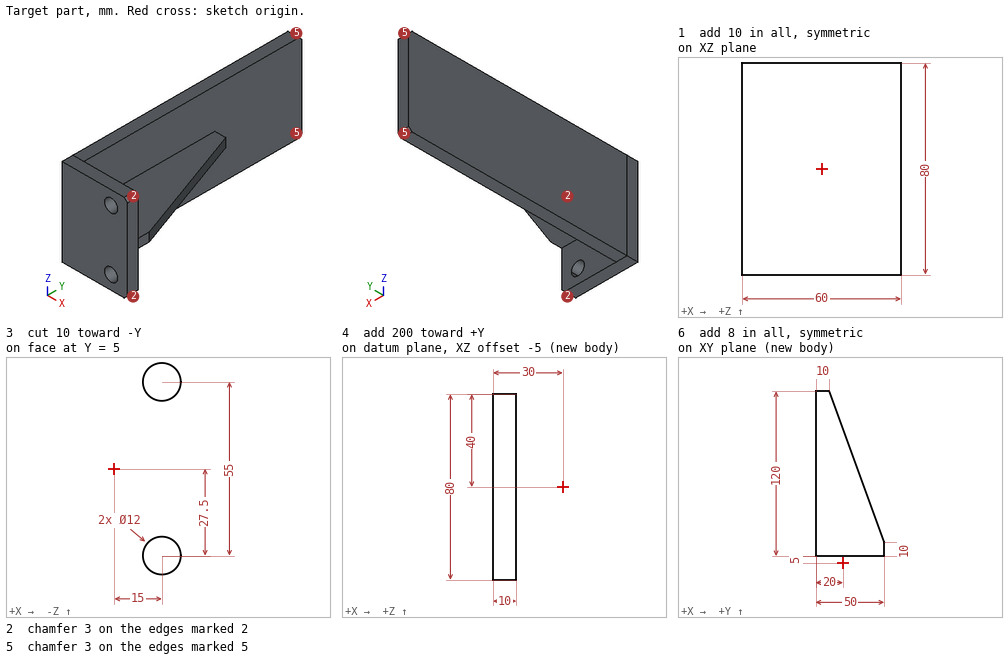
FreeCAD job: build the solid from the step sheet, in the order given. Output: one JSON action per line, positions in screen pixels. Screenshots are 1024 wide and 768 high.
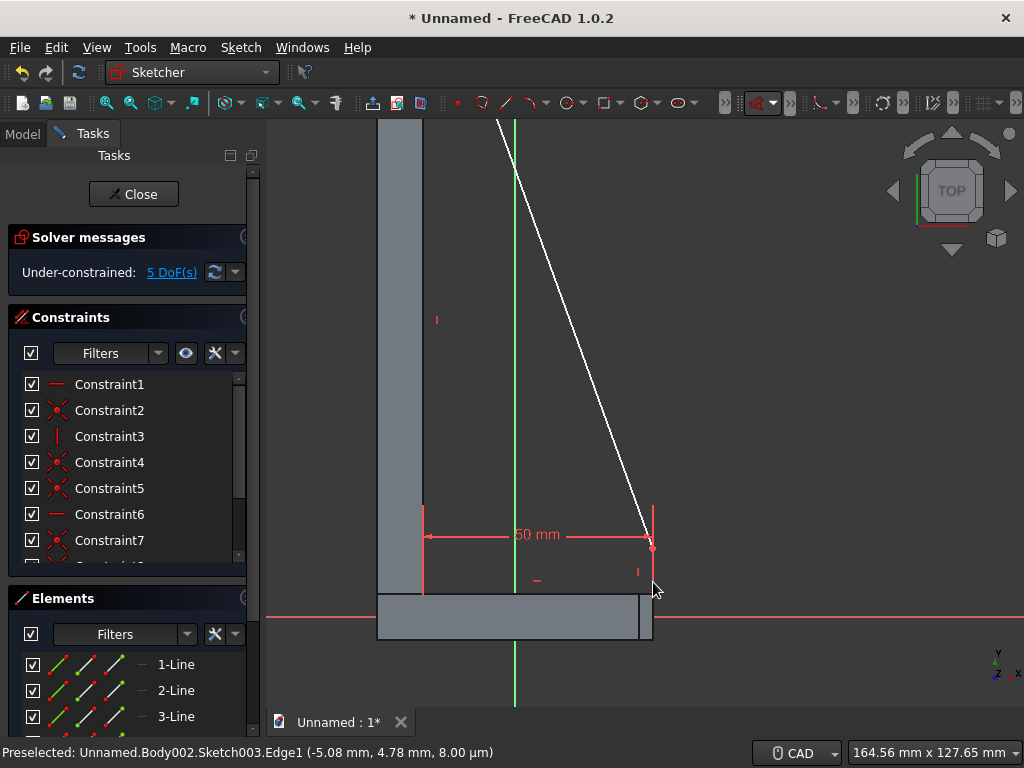
{"action": "left_click", "coordinate": [653, 581]}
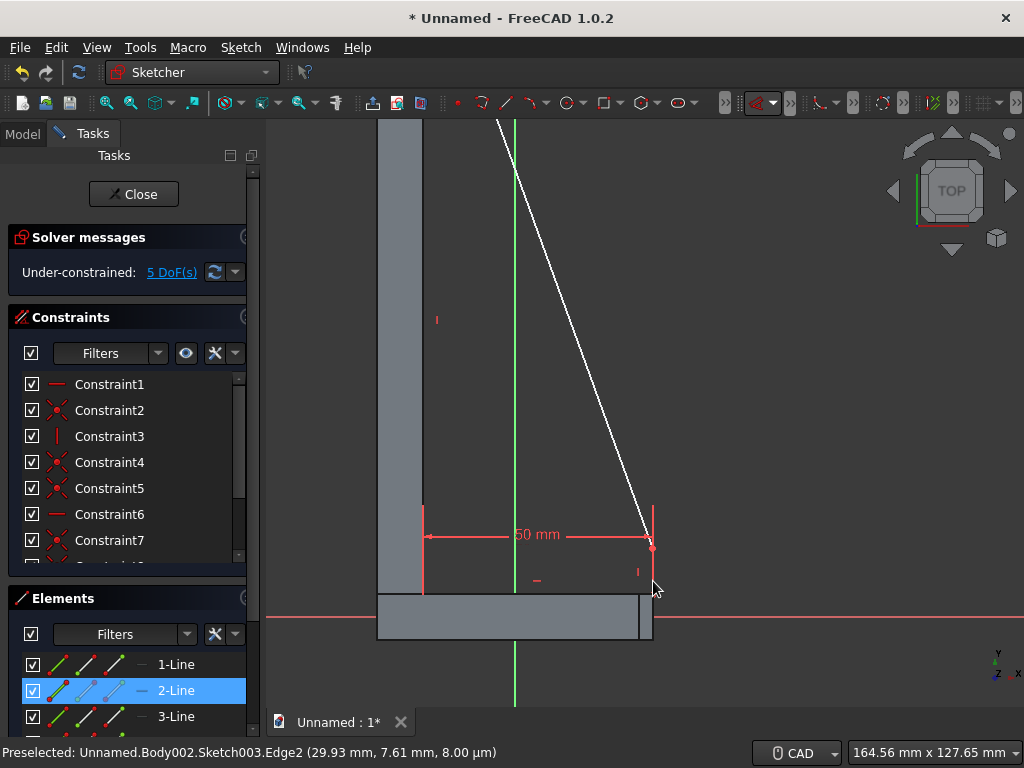
{"action": "left_click", "coordinate": [776, 104]}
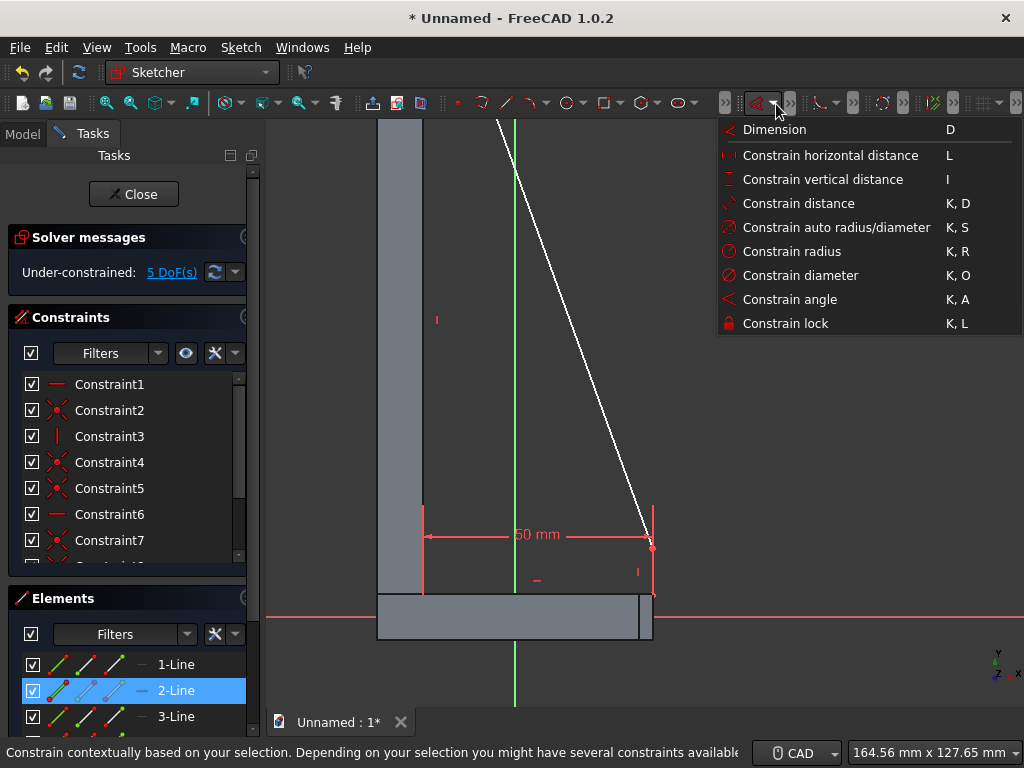
{"action": "left_click", "coordinate": [870, 179]}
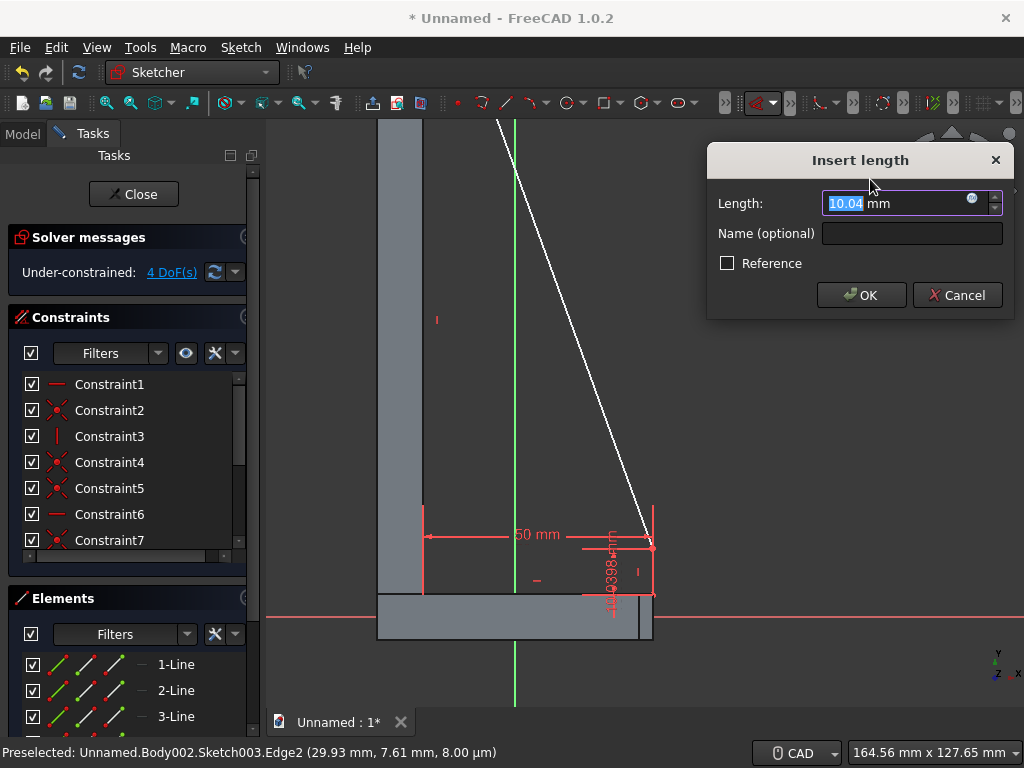
{"action": "type", "text": "10"}
{"action": "key", "text": "Return"}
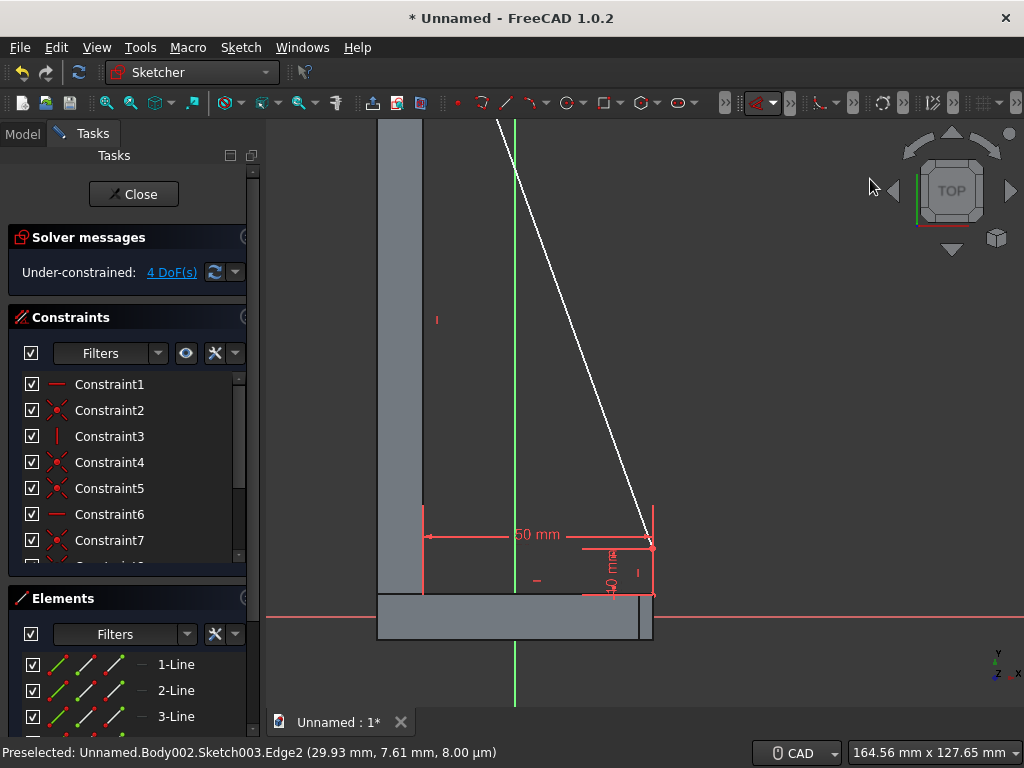
{"action": "scroll", "coordinate": [655, 583], "scroll_direction": "down", "scroll_amount": 2}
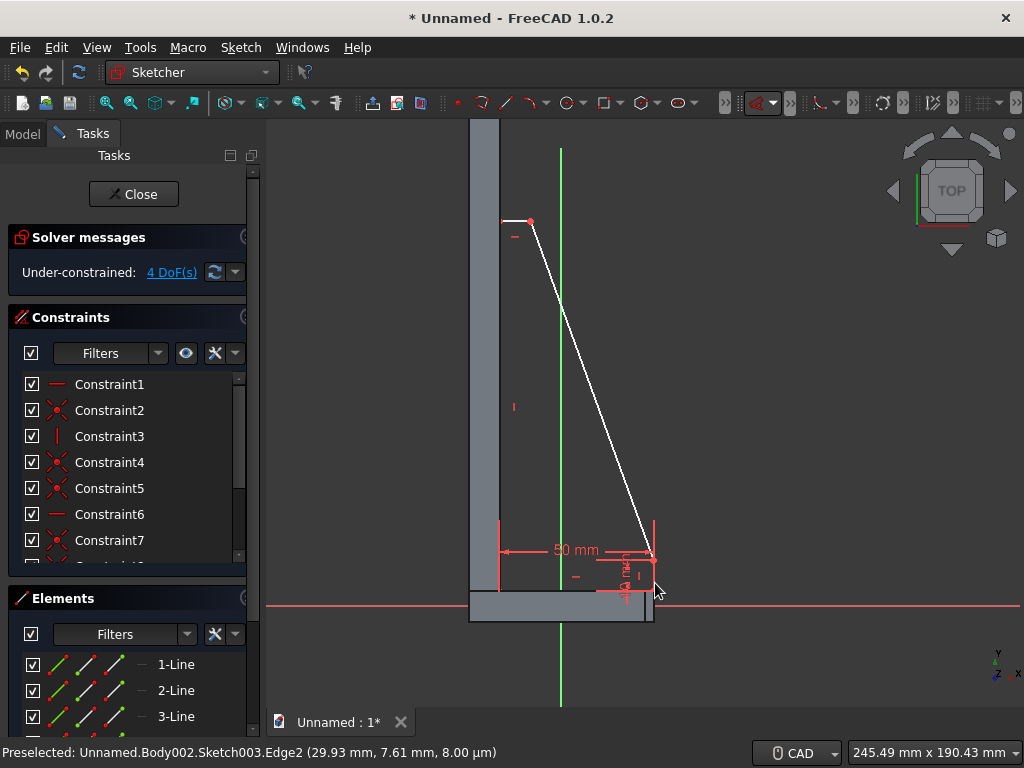
{"action": "scroll", "coordinate": [521, 221], "scroll_direction": "up", "scroll_amount": 2}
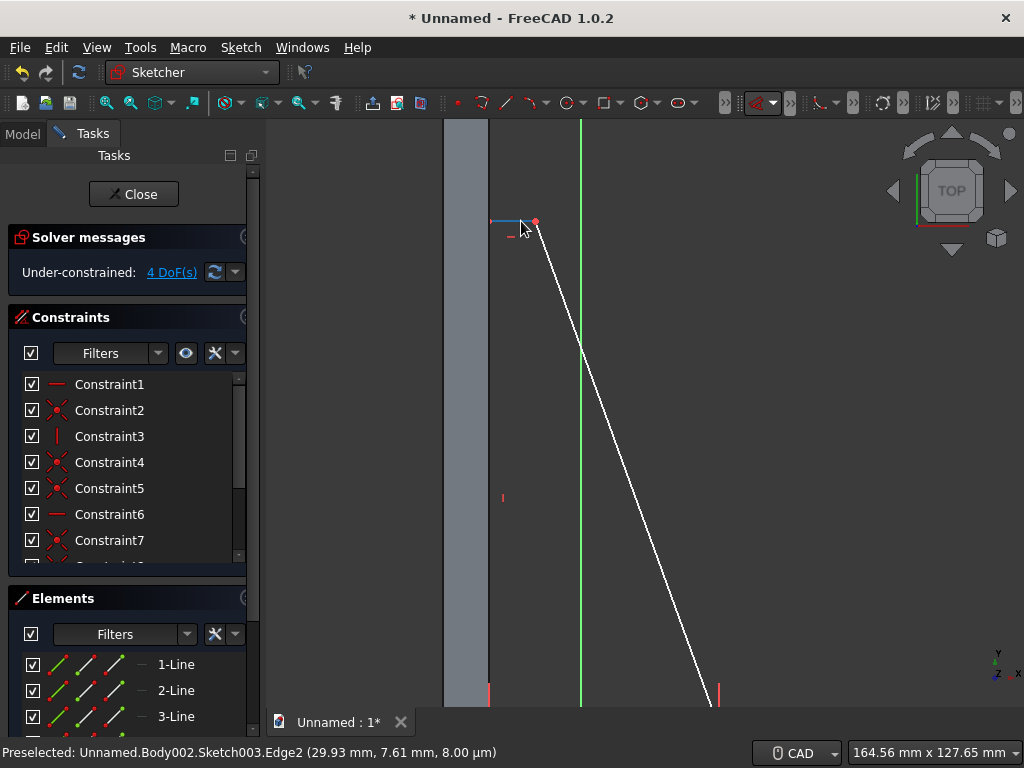
{"action": "left_click", "coordinate": [521, 221]}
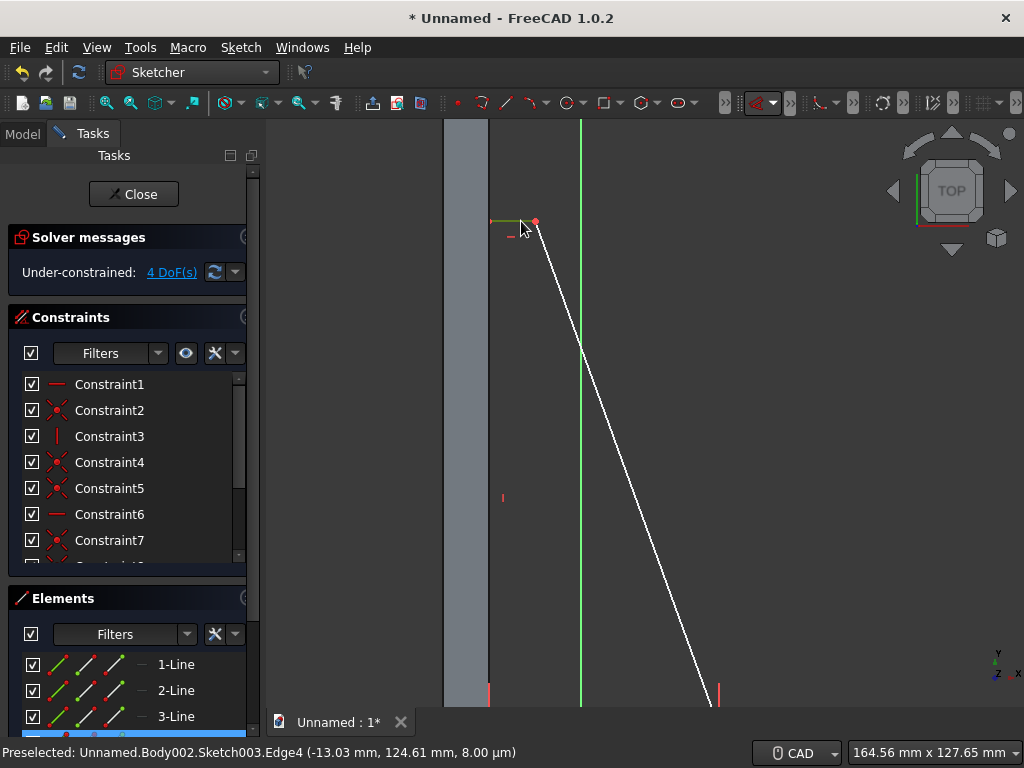
{"action": "left_click", "coordinate": [776, 104]}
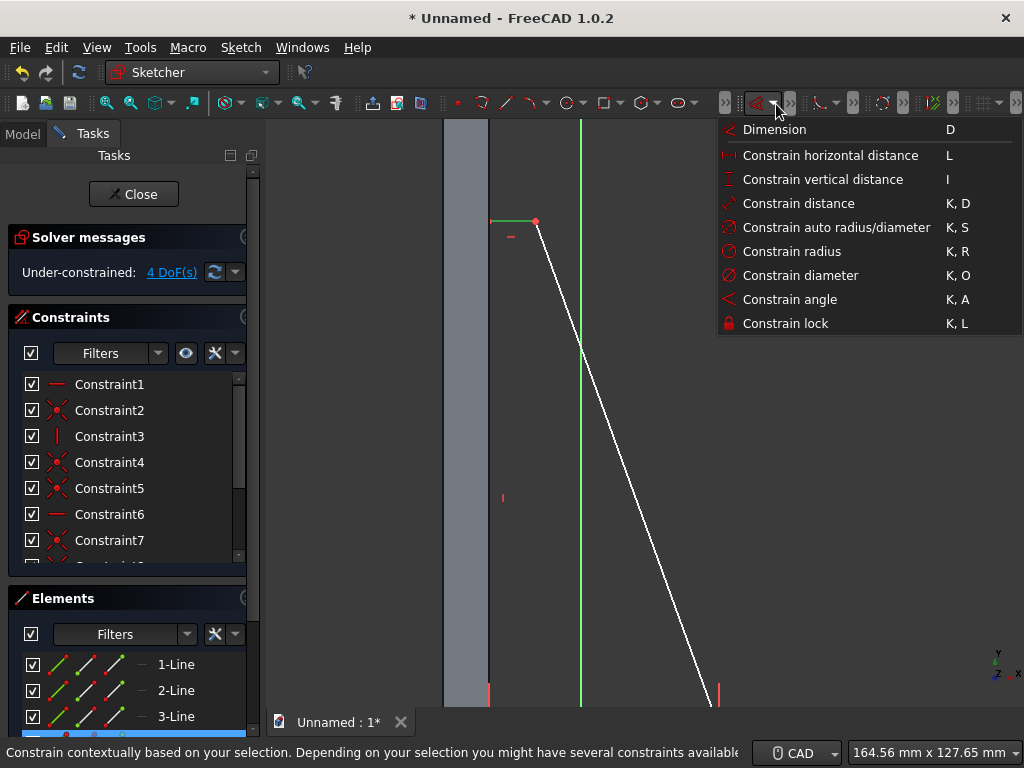
{"action": "left_click", "coordinate": [870, 155]}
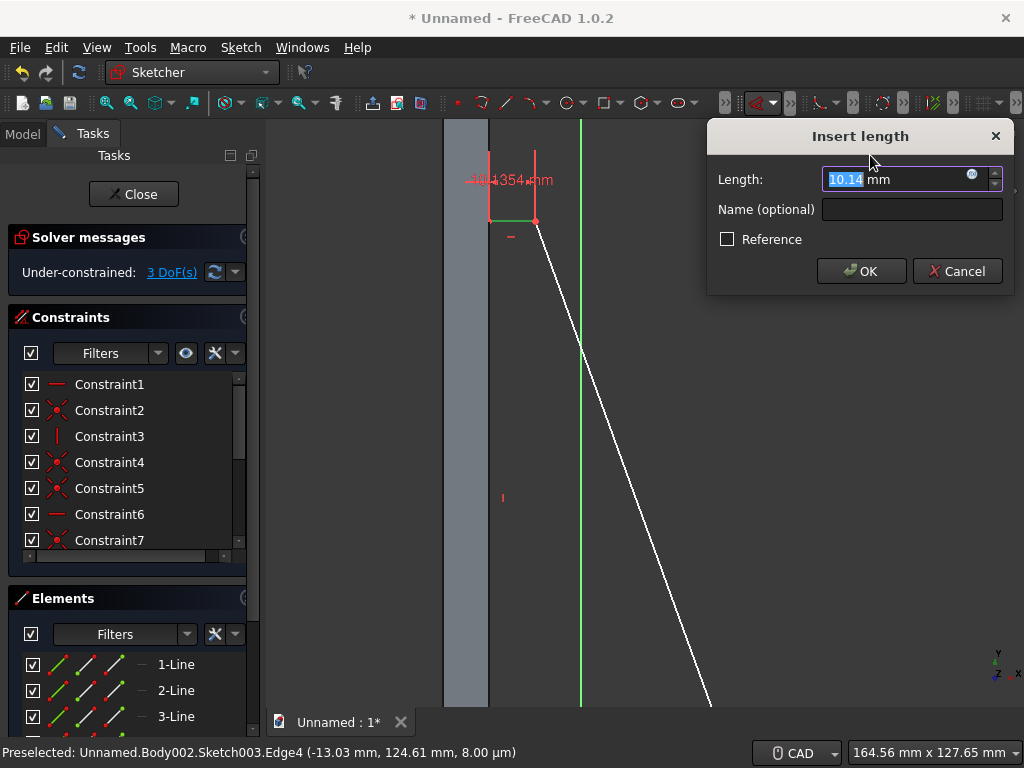
{"action": "type", "text": "10"}
{"action": "key", "text": "Return"}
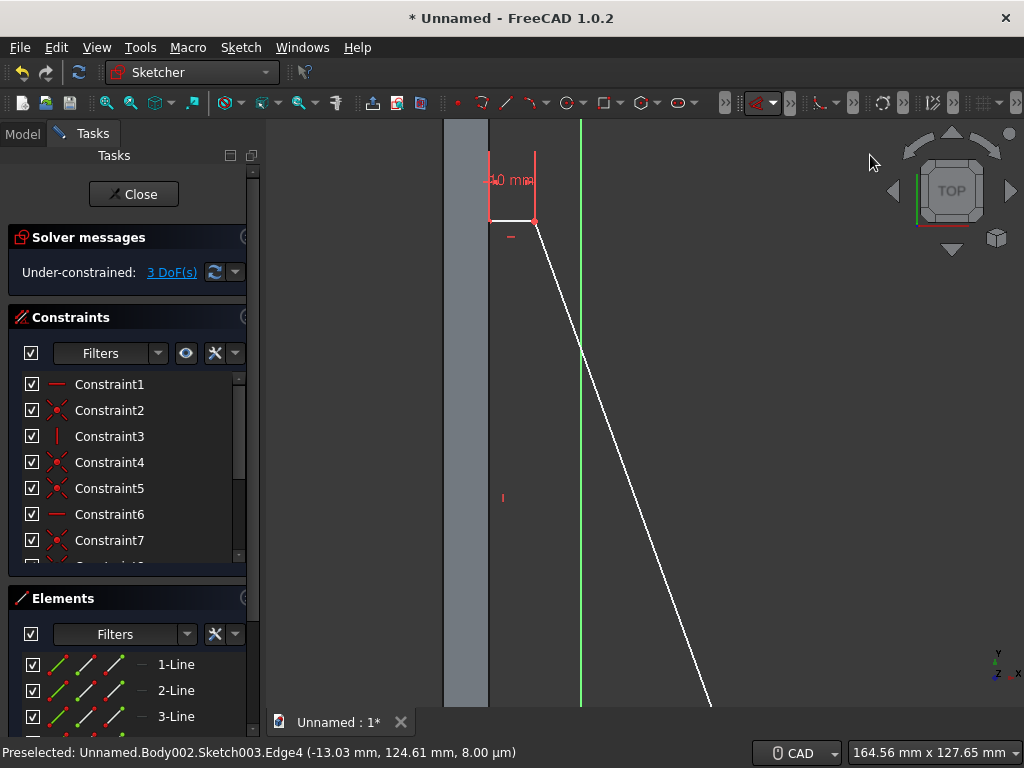
{"action": "scroll", "coordinate": [520, 221], "scroll_direction": "down", "scroll_amount": 2}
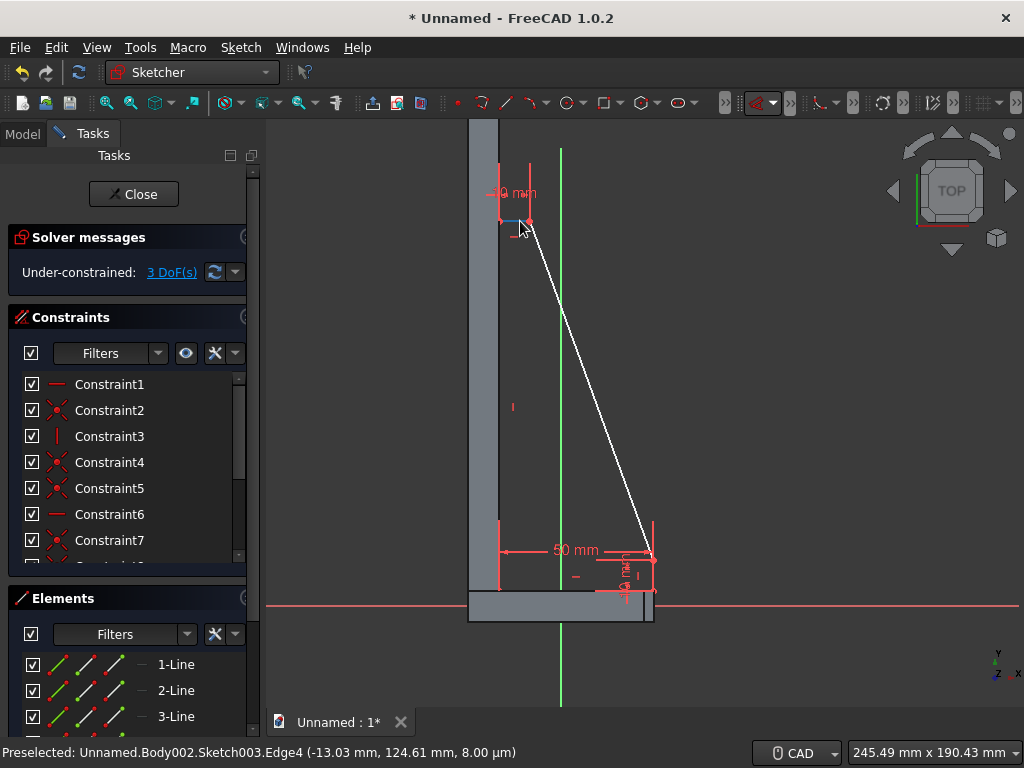
{"action": "scroll", "coordinate": [499, 591], "scroll_direction": "up", "scroll_amount": 5}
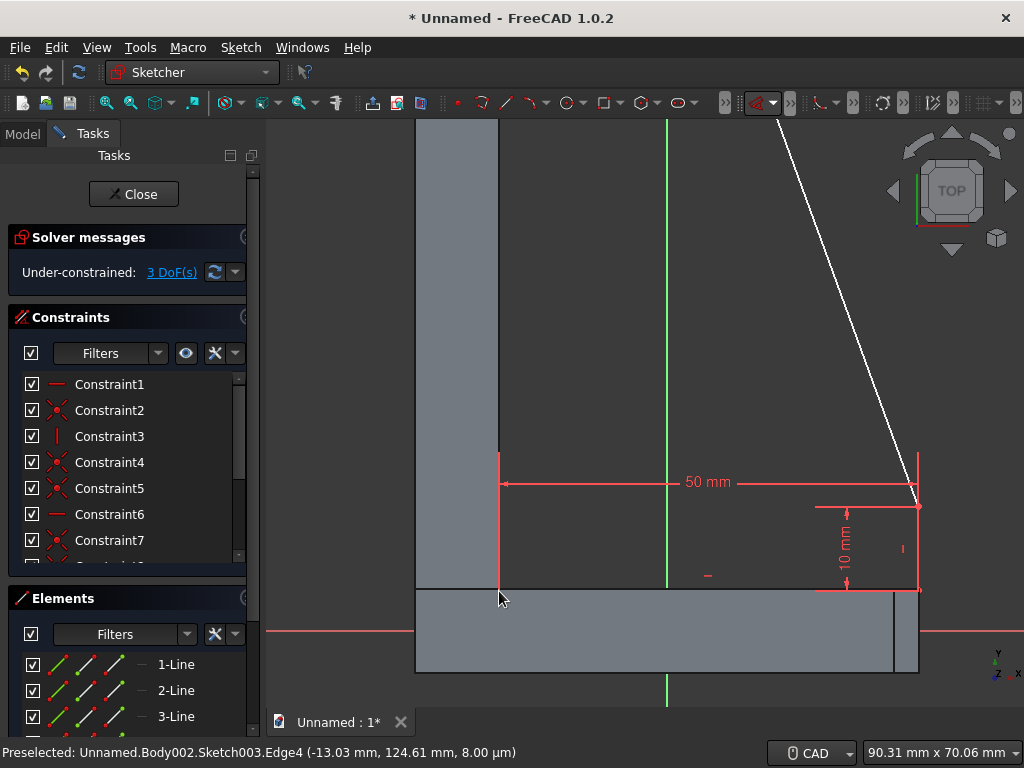
{"action": "left_click", "coordinate": [499, 591]}